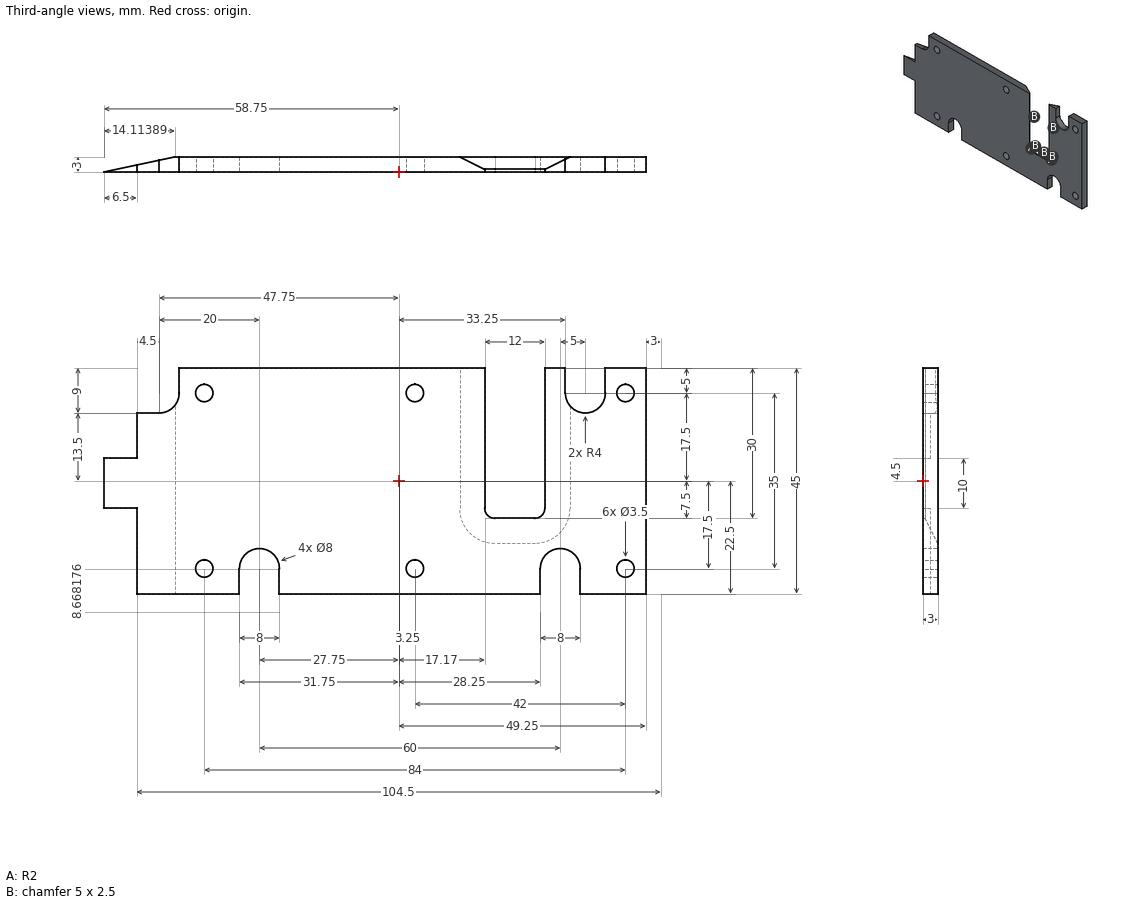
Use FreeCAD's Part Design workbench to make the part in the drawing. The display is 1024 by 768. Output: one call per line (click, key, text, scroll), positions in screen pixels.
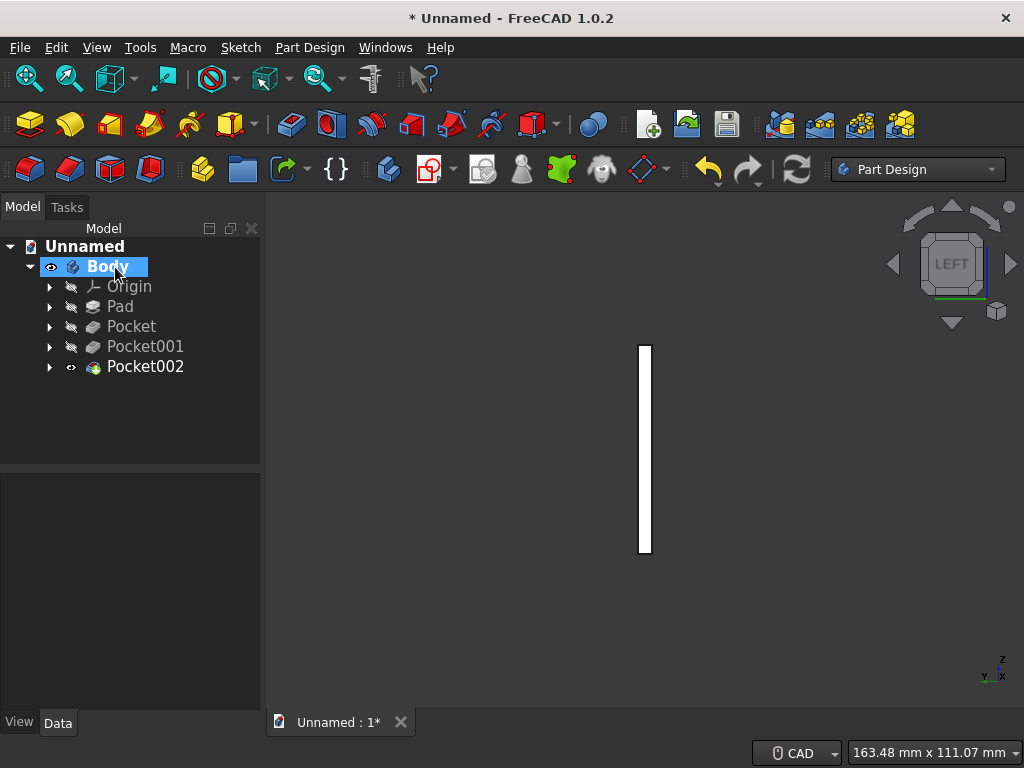
scroll(645, 448, up, 3)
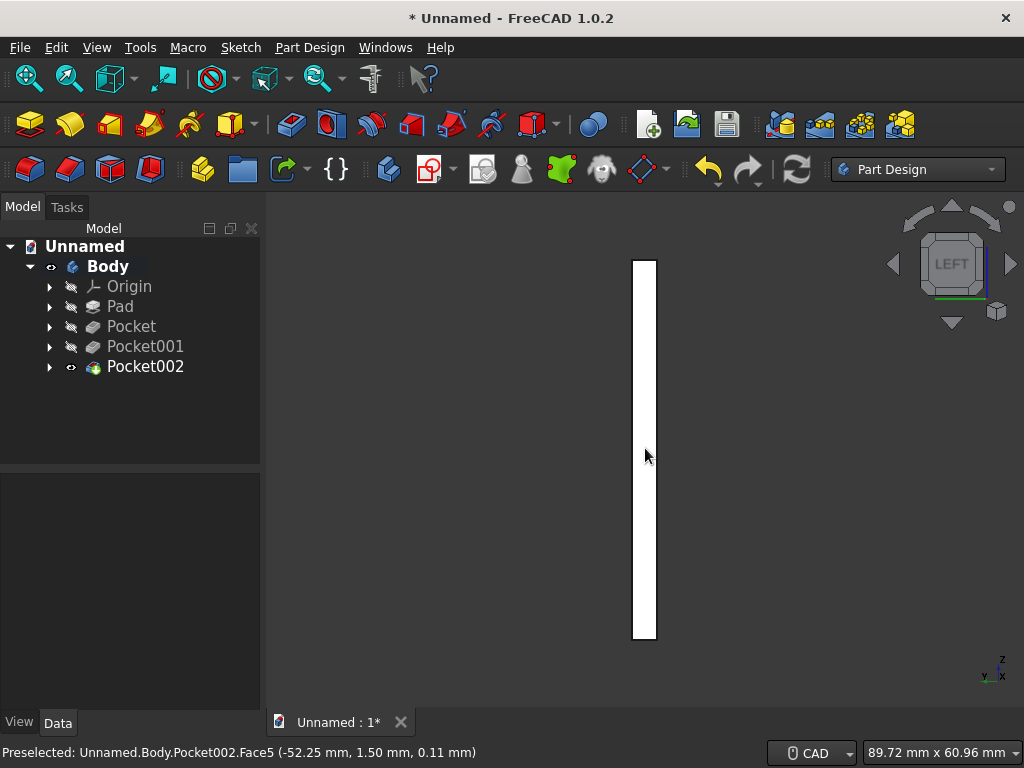
click(645, 449)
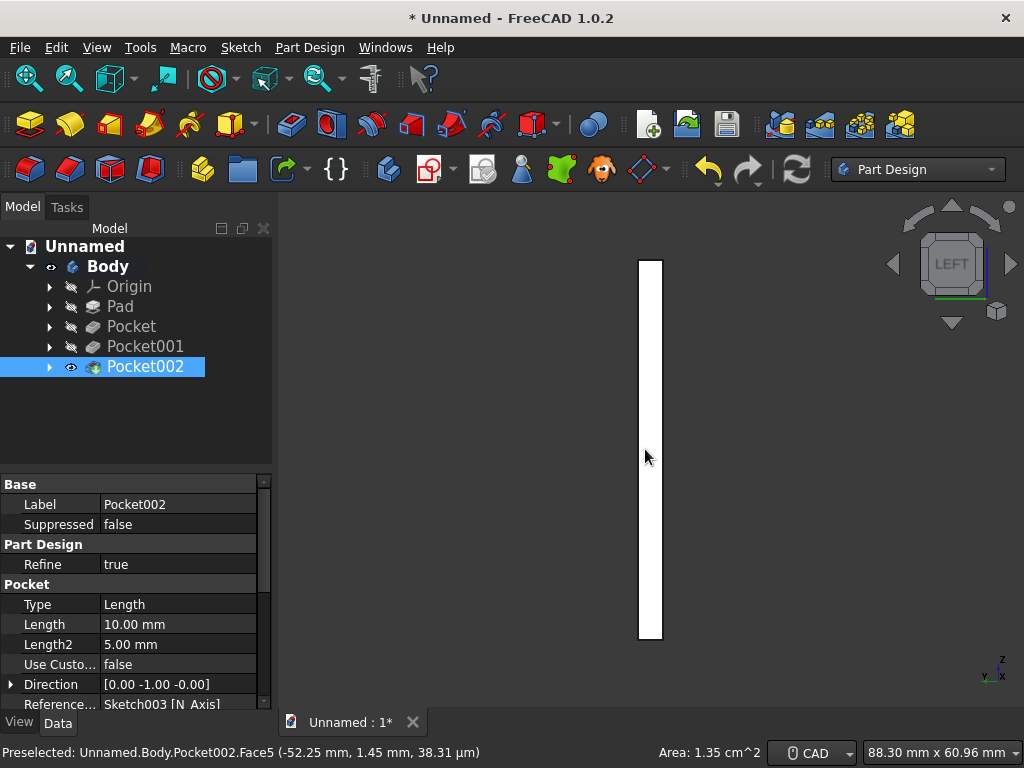
click(430, 170)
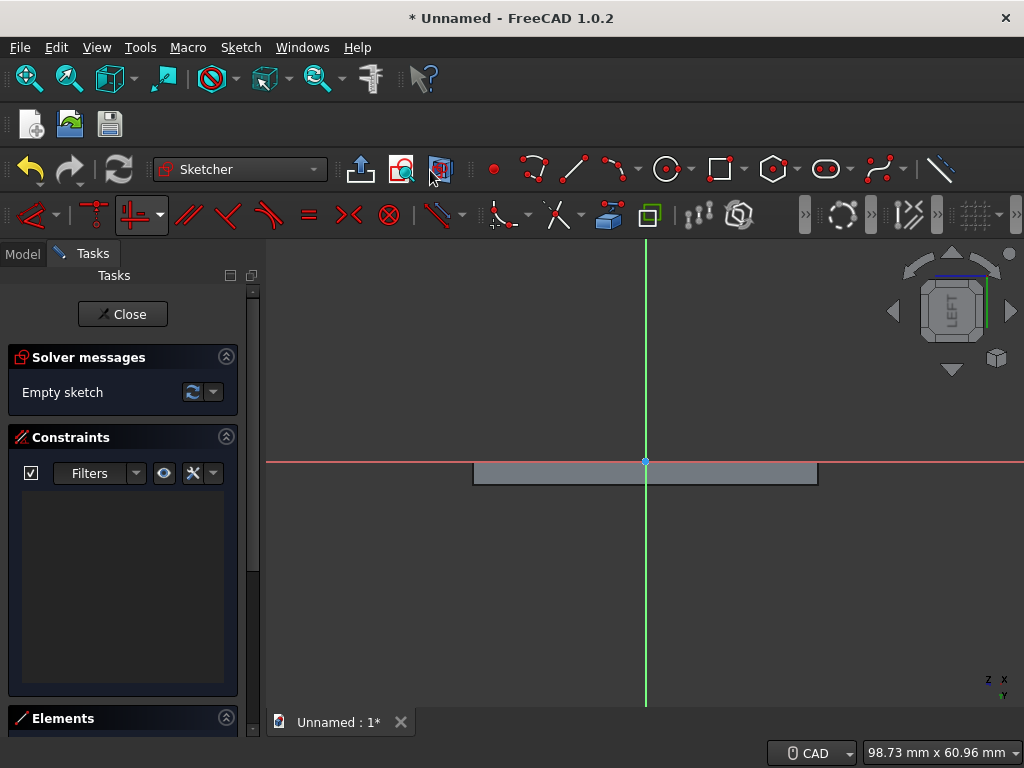
scroll(668, 473, up, 8)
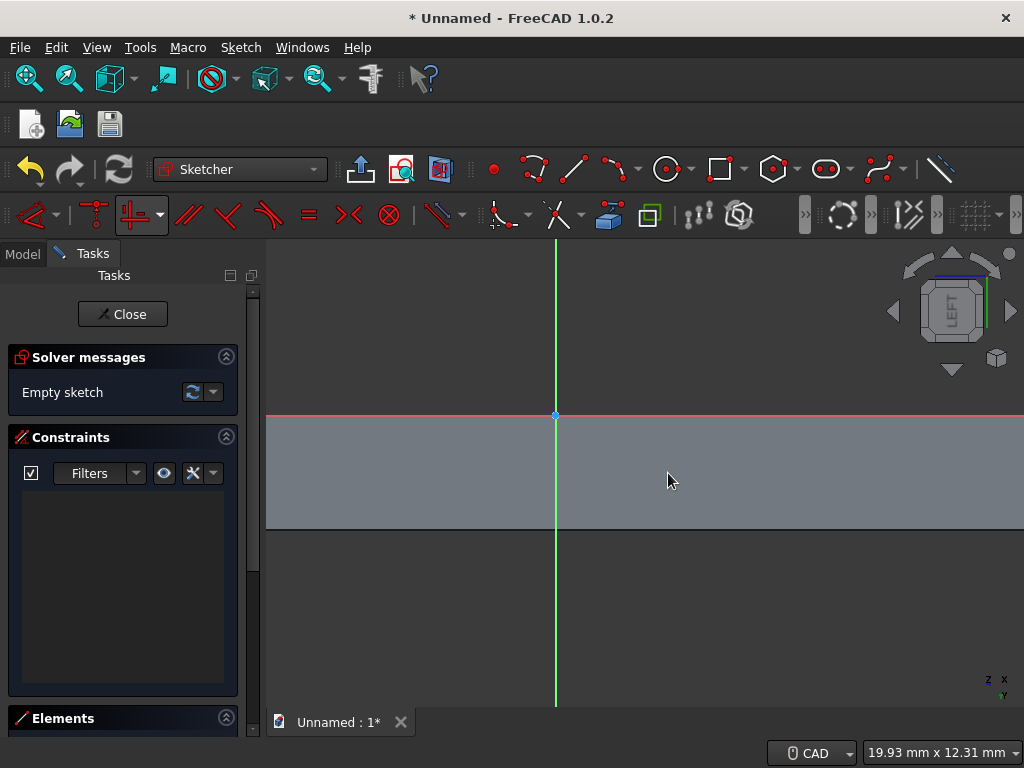
key(g)
key(r)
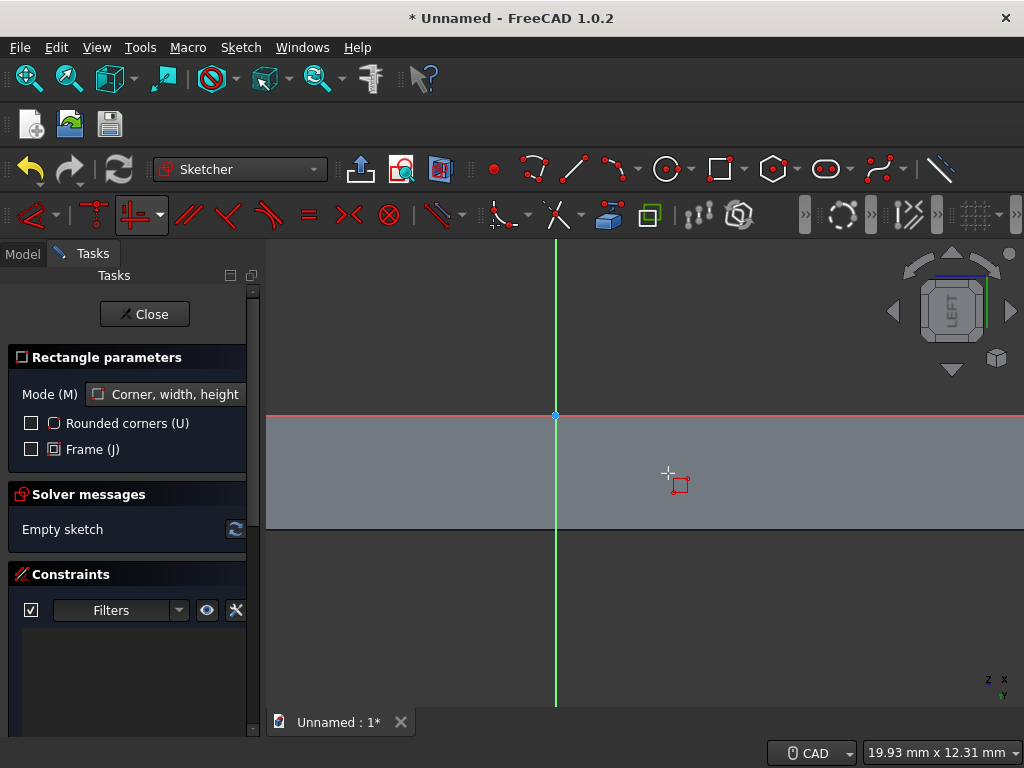
click(385, 416)
move(765, 530)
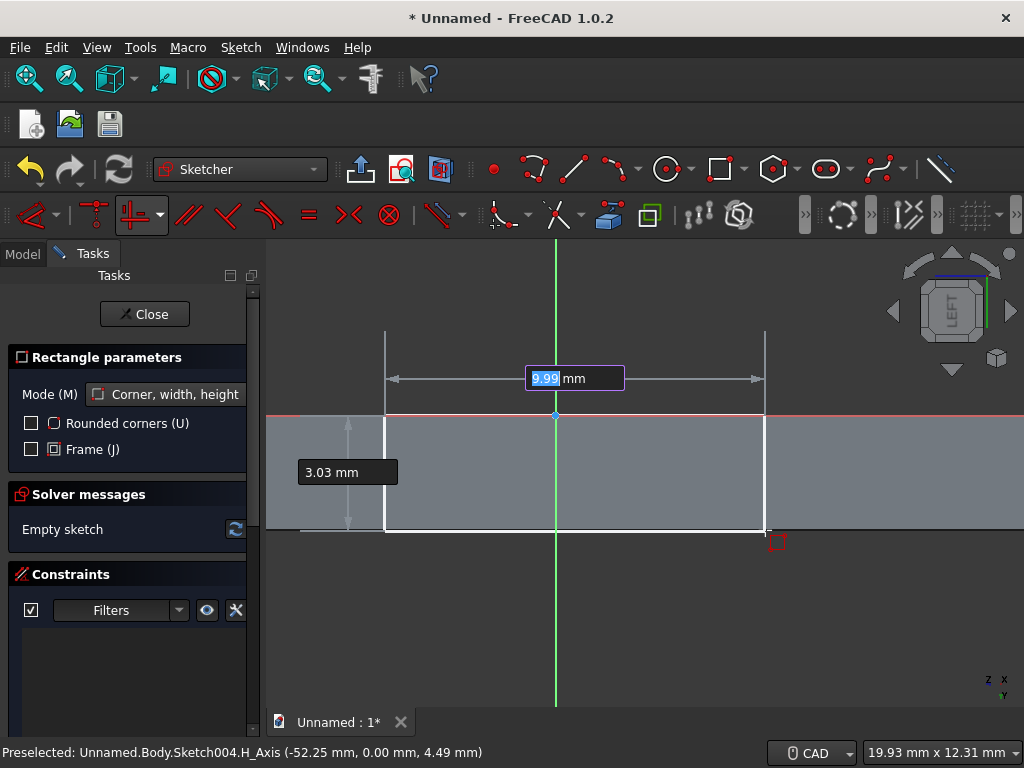
text(10)
key(Tab)
text(3)
key(Return)
key(Escape)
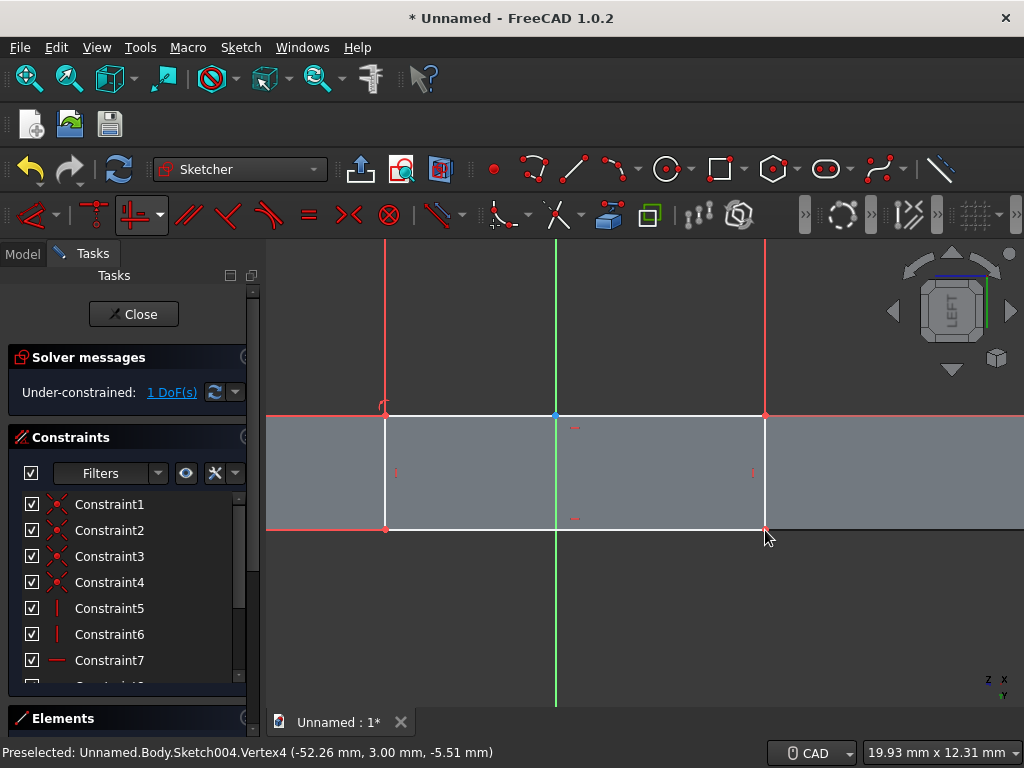
key(d)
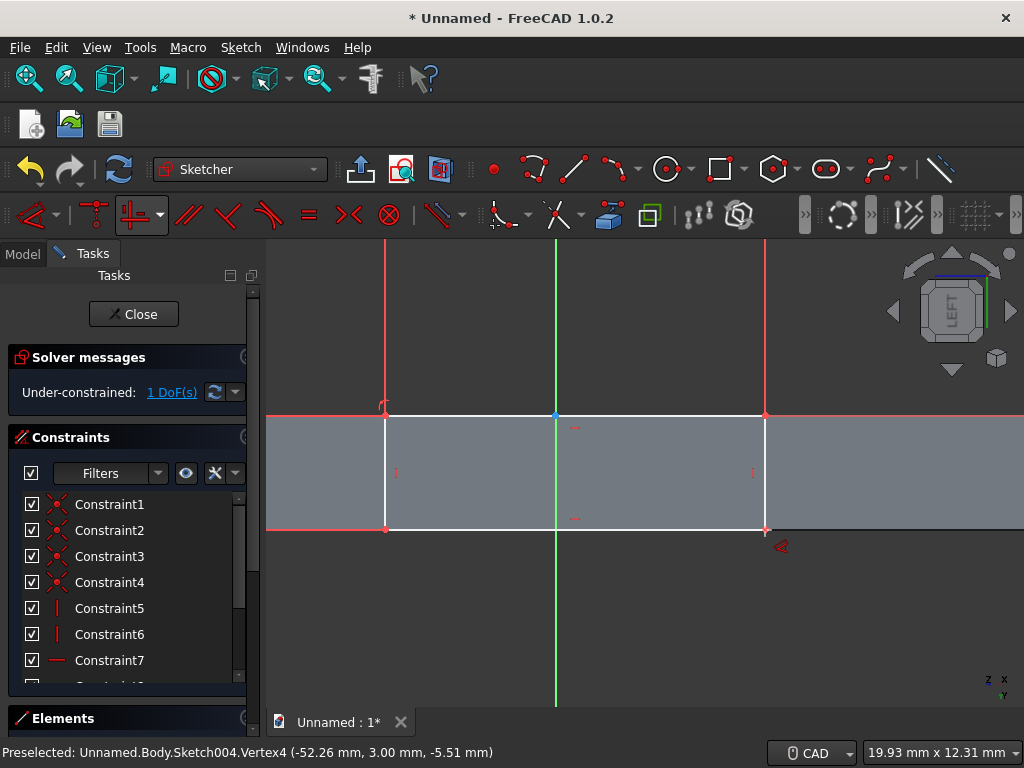
click(385, 416)
click(470, 382)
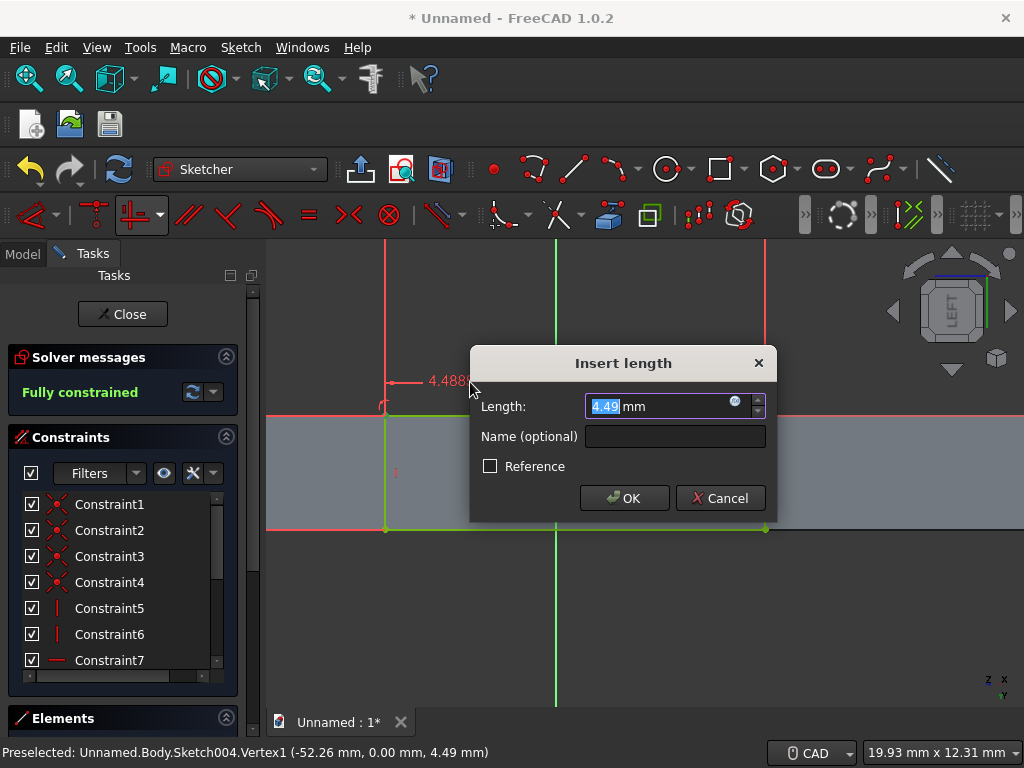
text(4.5)
key(Return)
key(Escape)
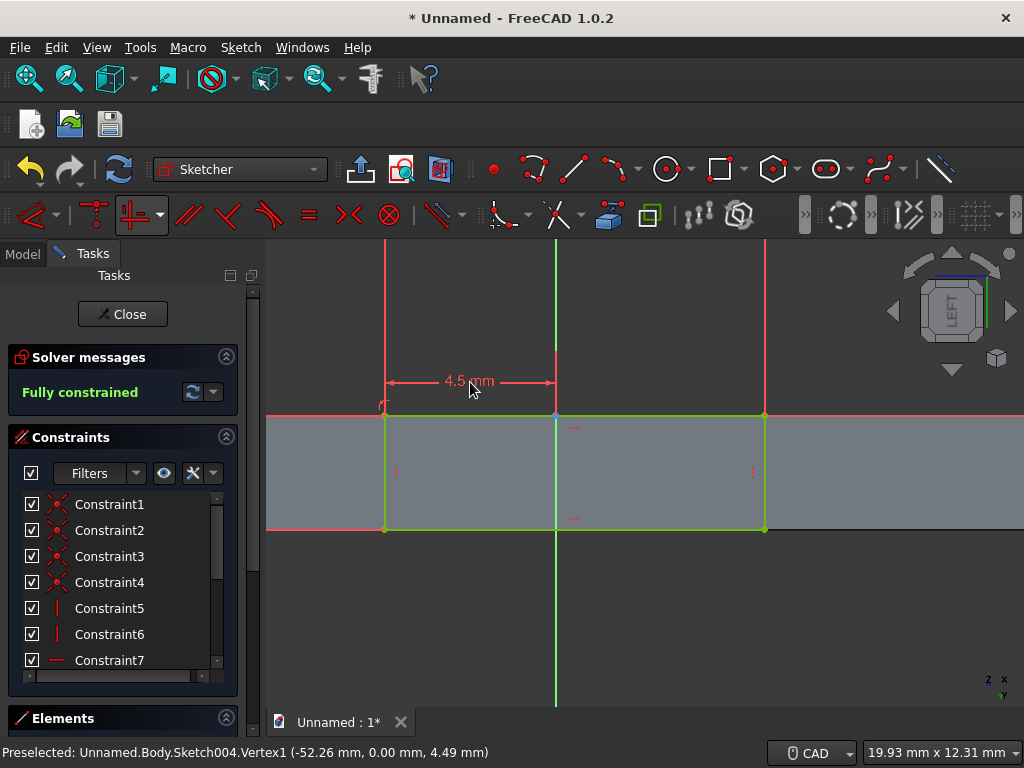
click(123, 314)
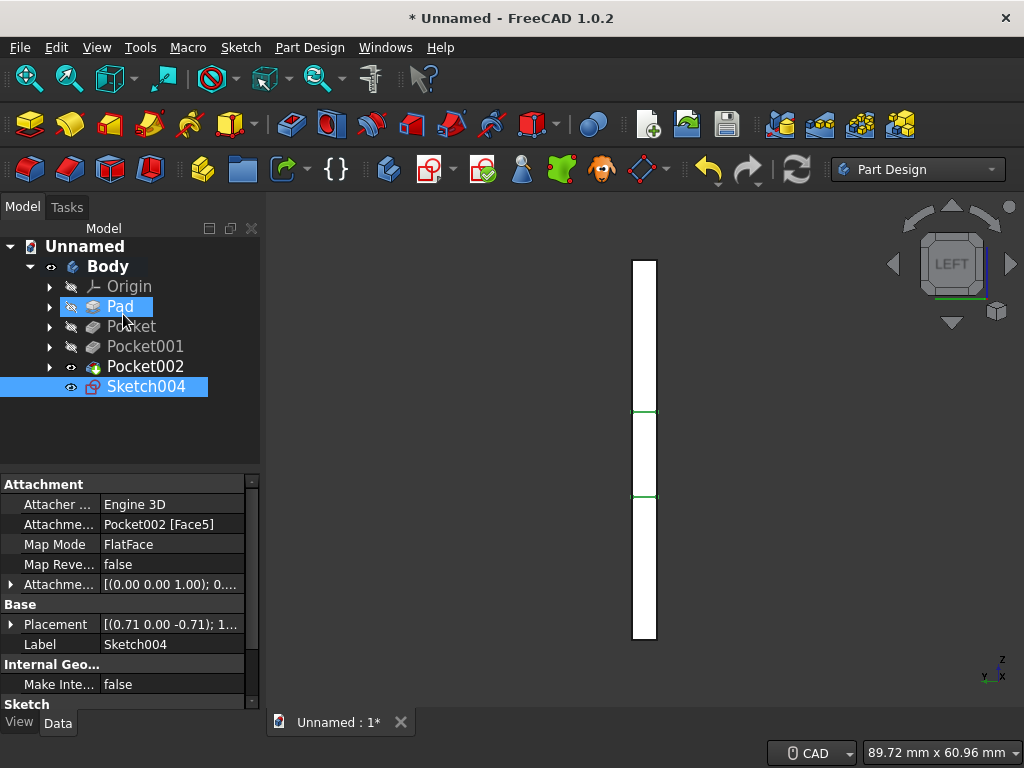
click(30, 124)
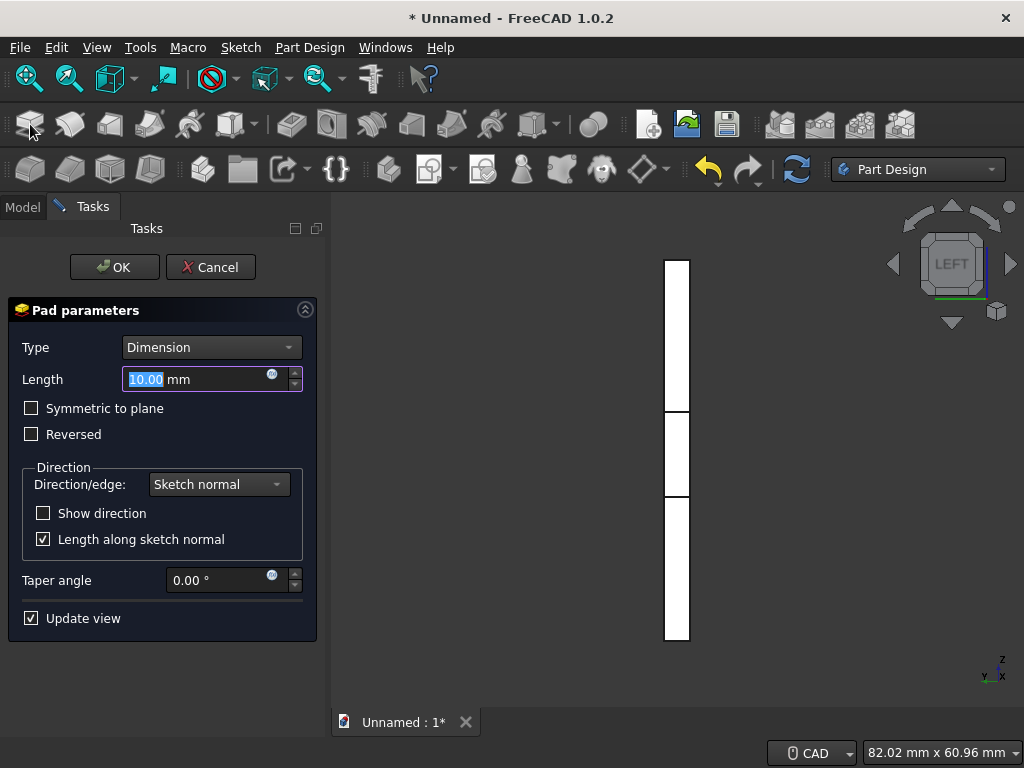
text(6.5)
key(Tab)